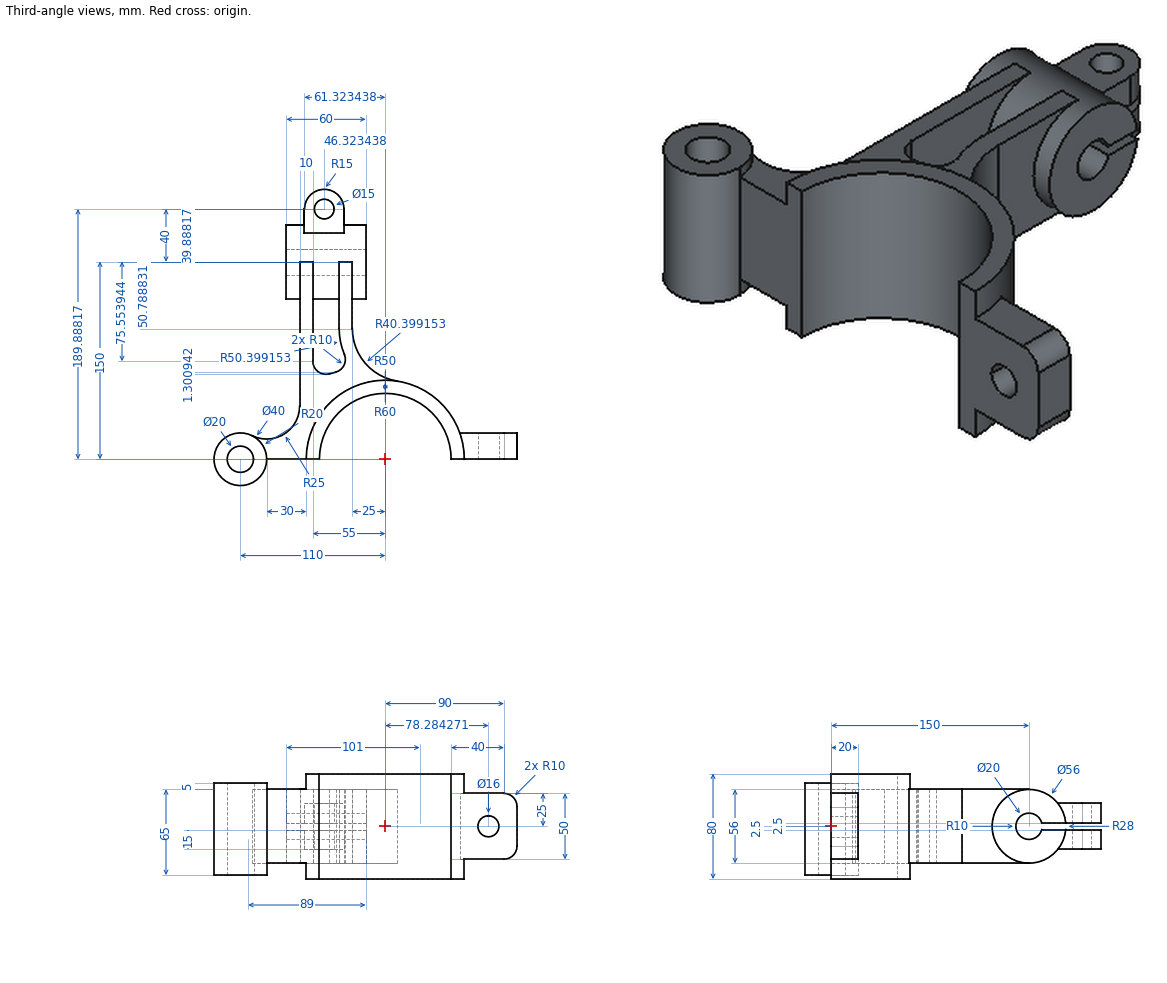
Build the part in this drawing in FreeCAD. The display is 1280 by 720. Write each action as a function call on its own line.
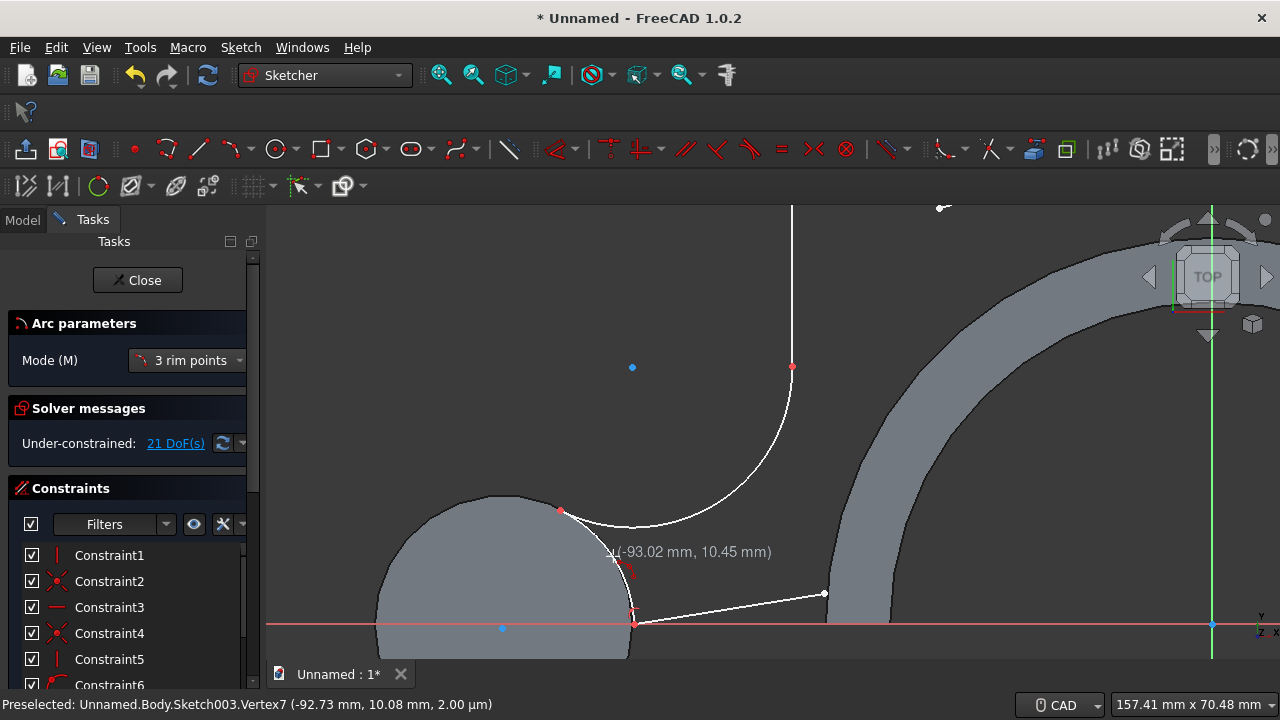
scroll(613, 557, down, 6)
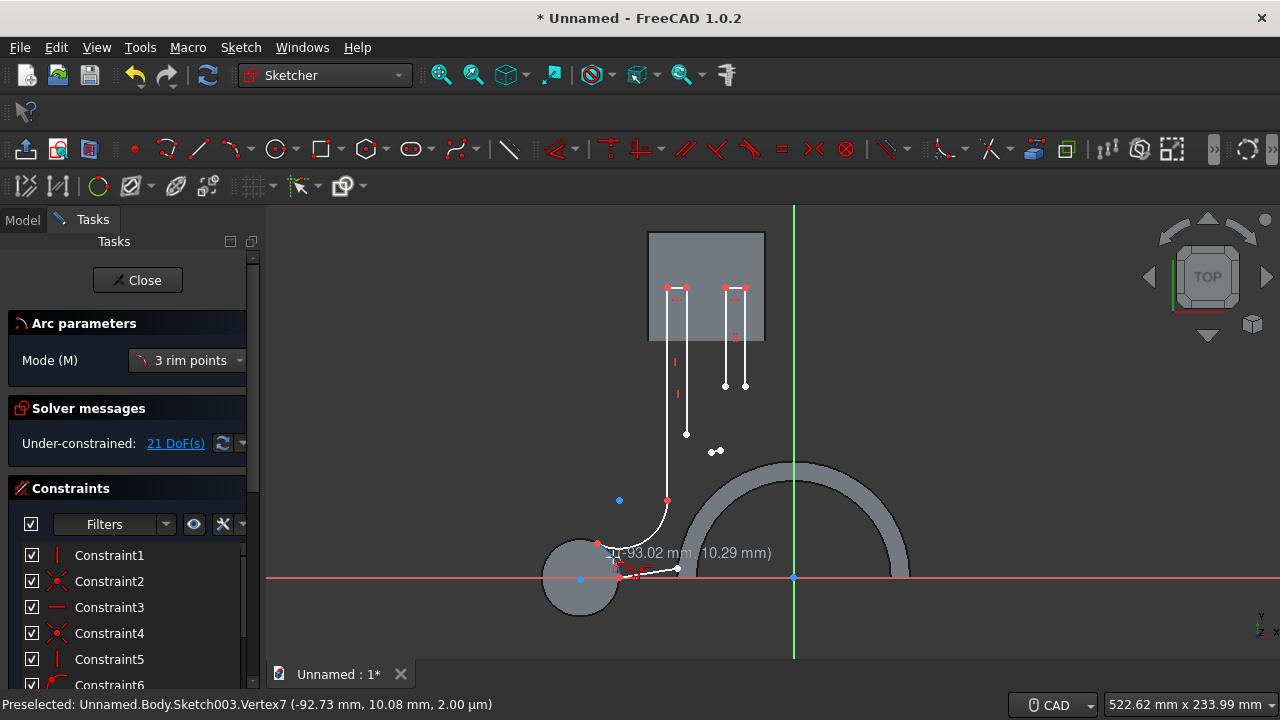
click(677, 569)
click(812, 463)
click(718, 489)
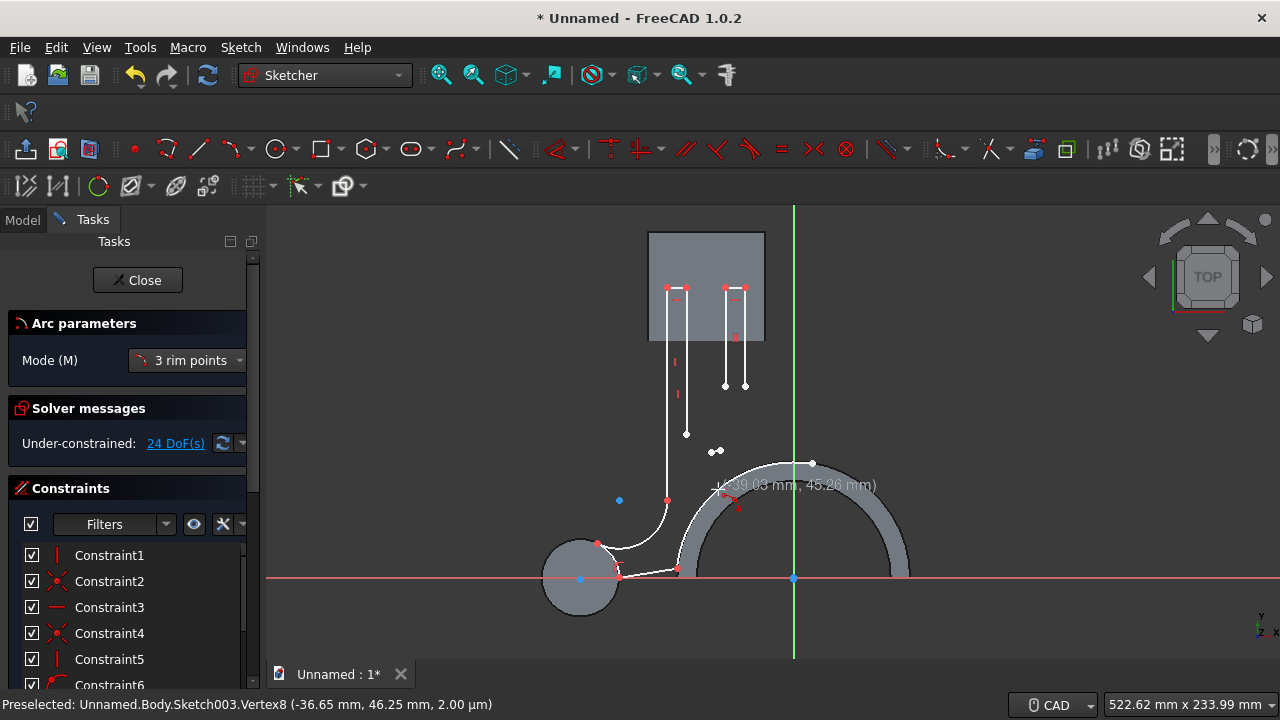
click(812, 464)
click(745, 387)
click(764, 436)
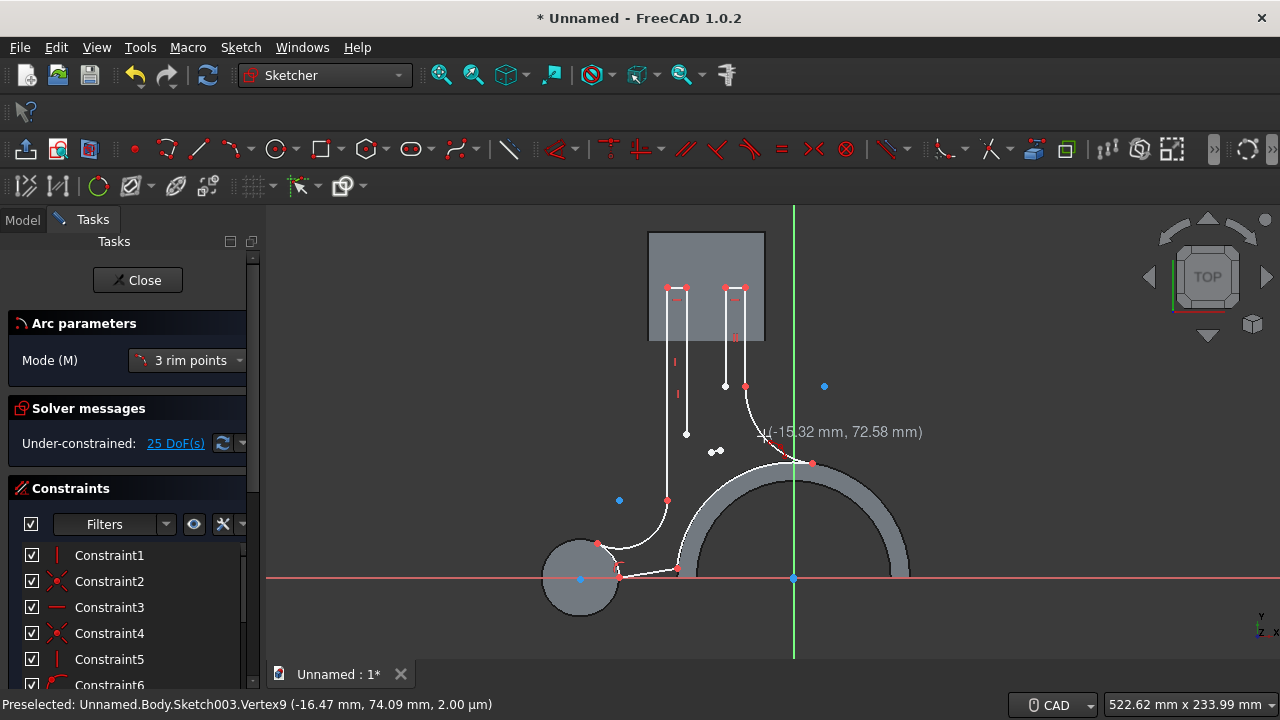
click(726, 387)
click(734, 423)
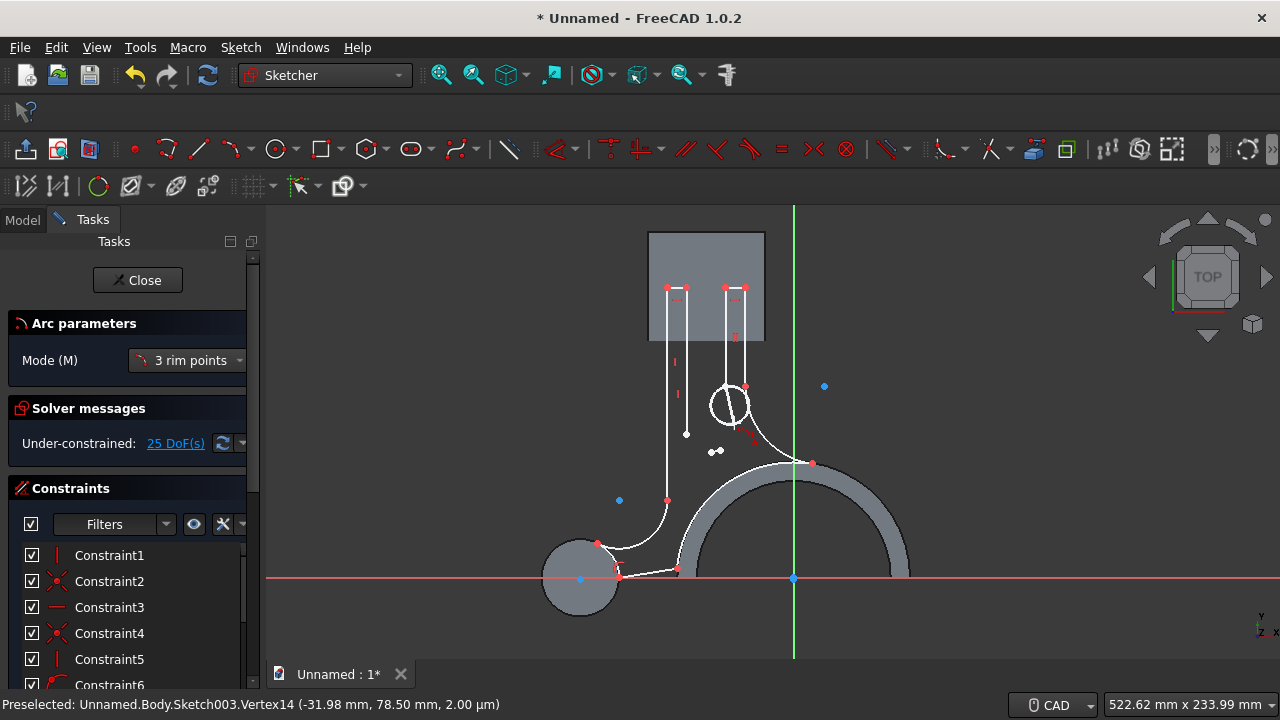
scroll(728, 405, up, 11)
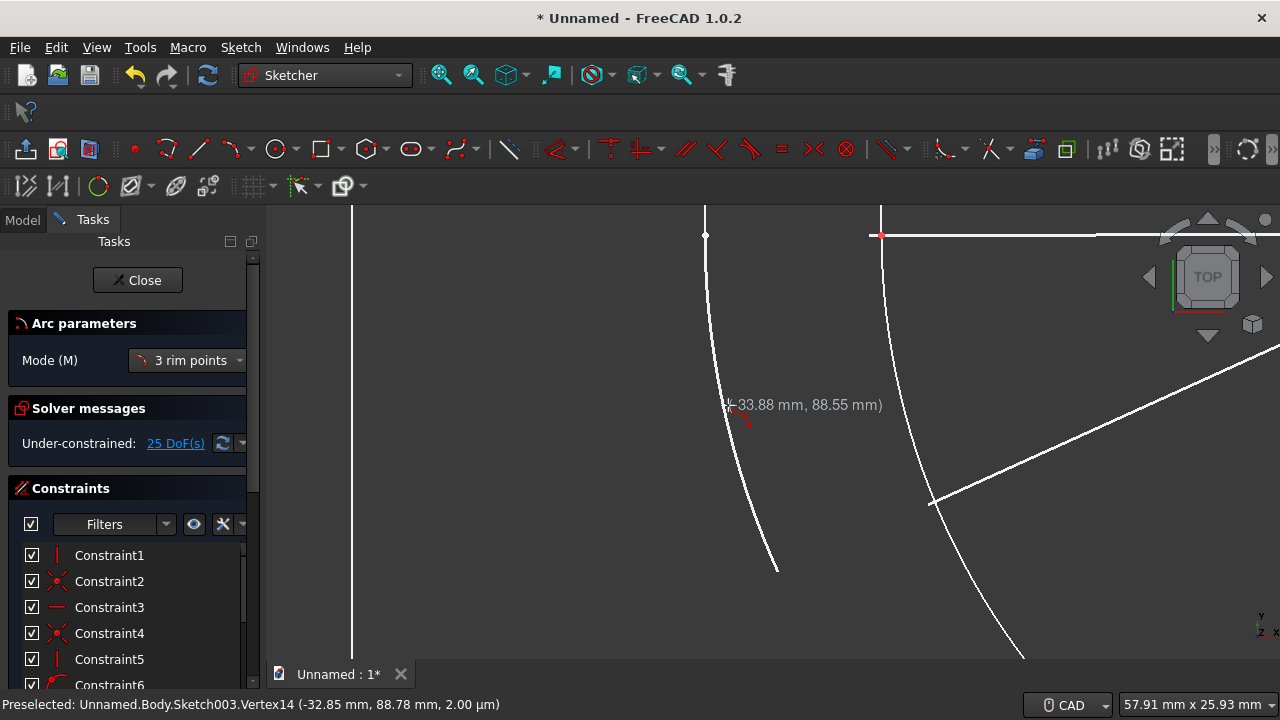
click(722, 399)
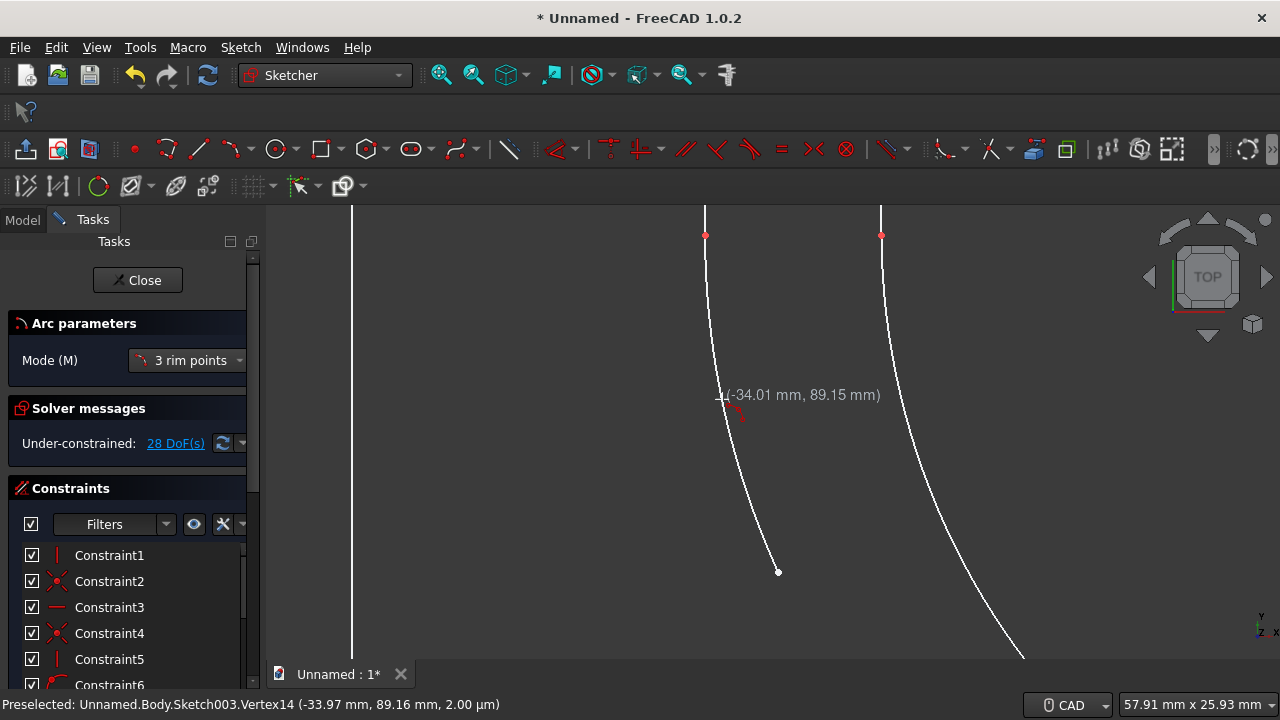
scroll(728, 405, down, 11)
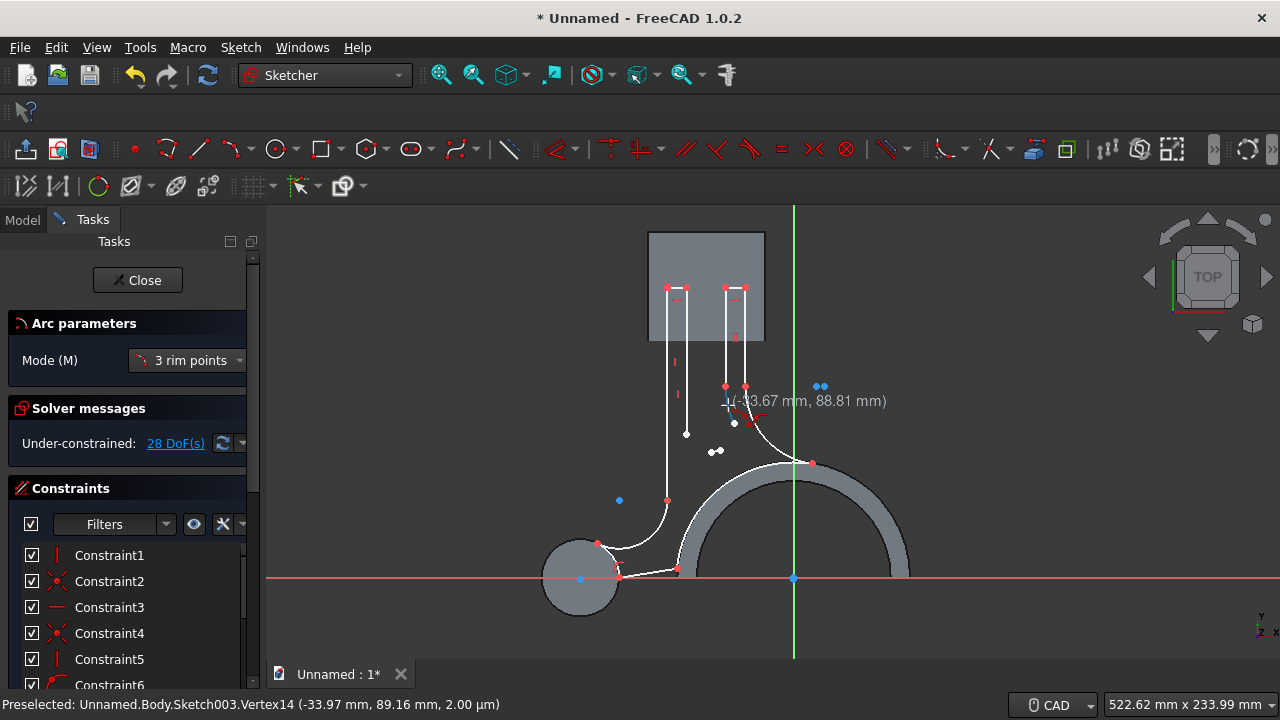
click(734, 424)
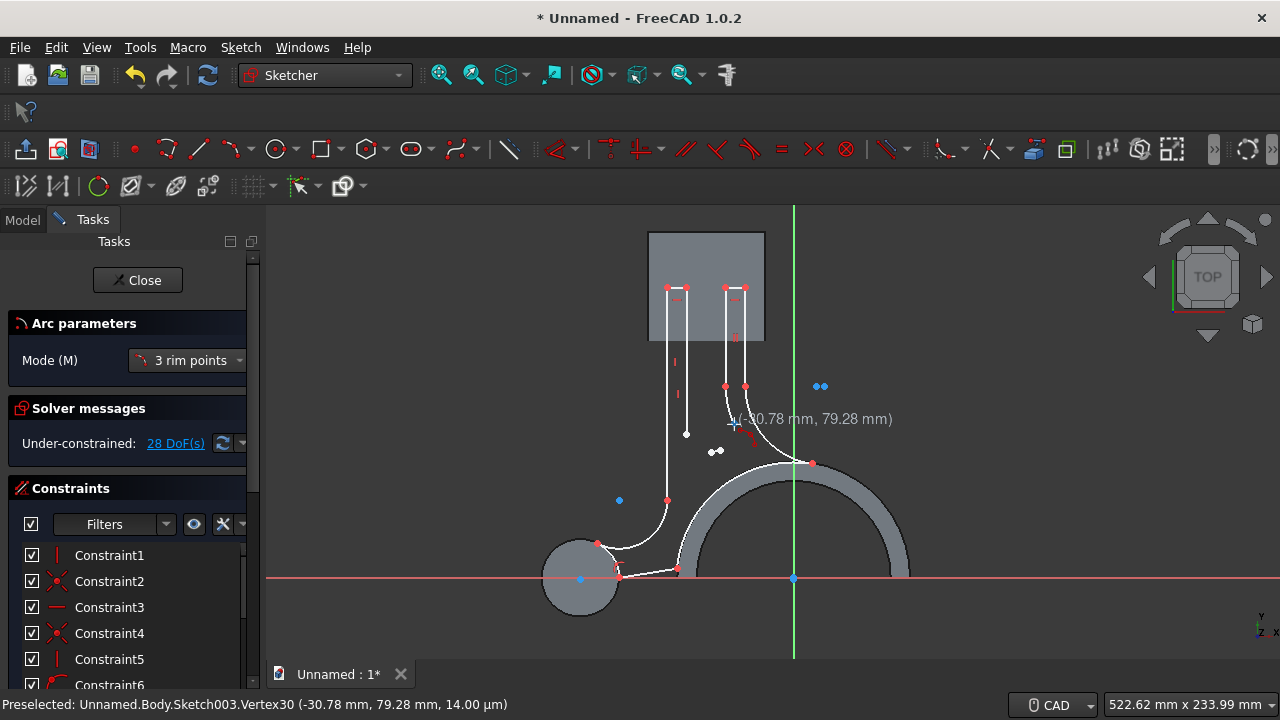
scroll(721, 450, up, 7)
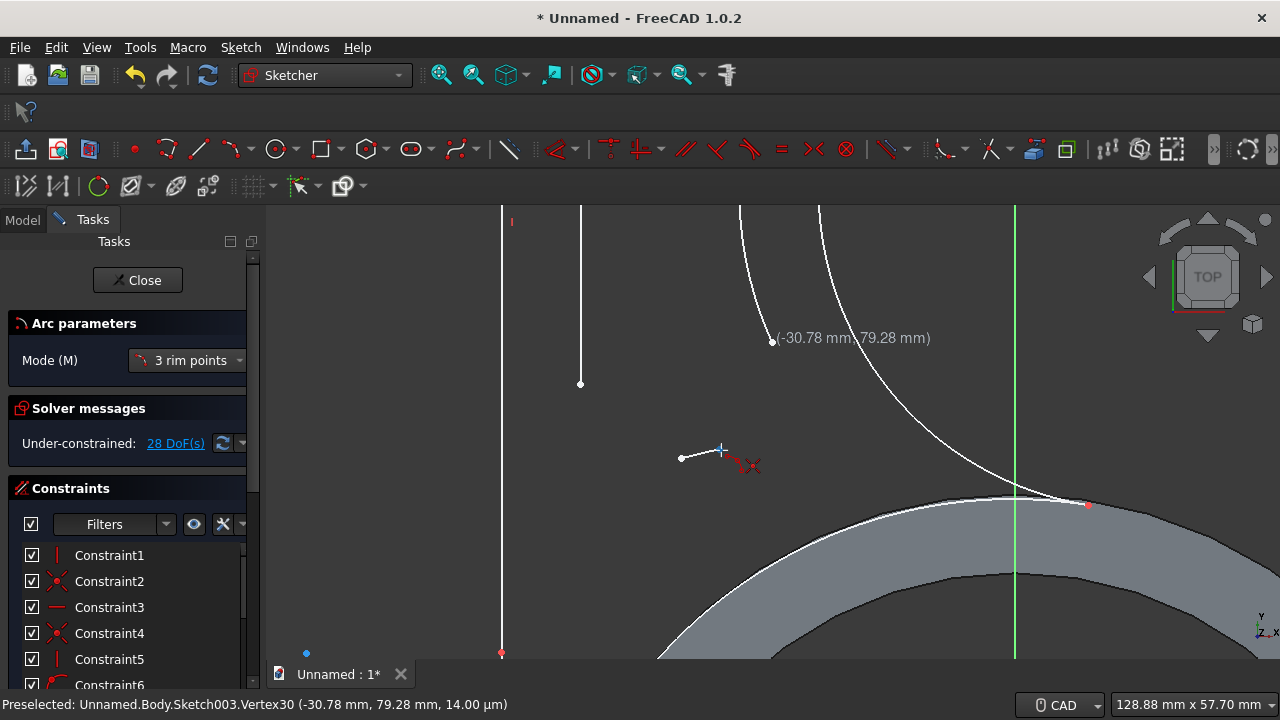
click(720, 449)
click(769, 405)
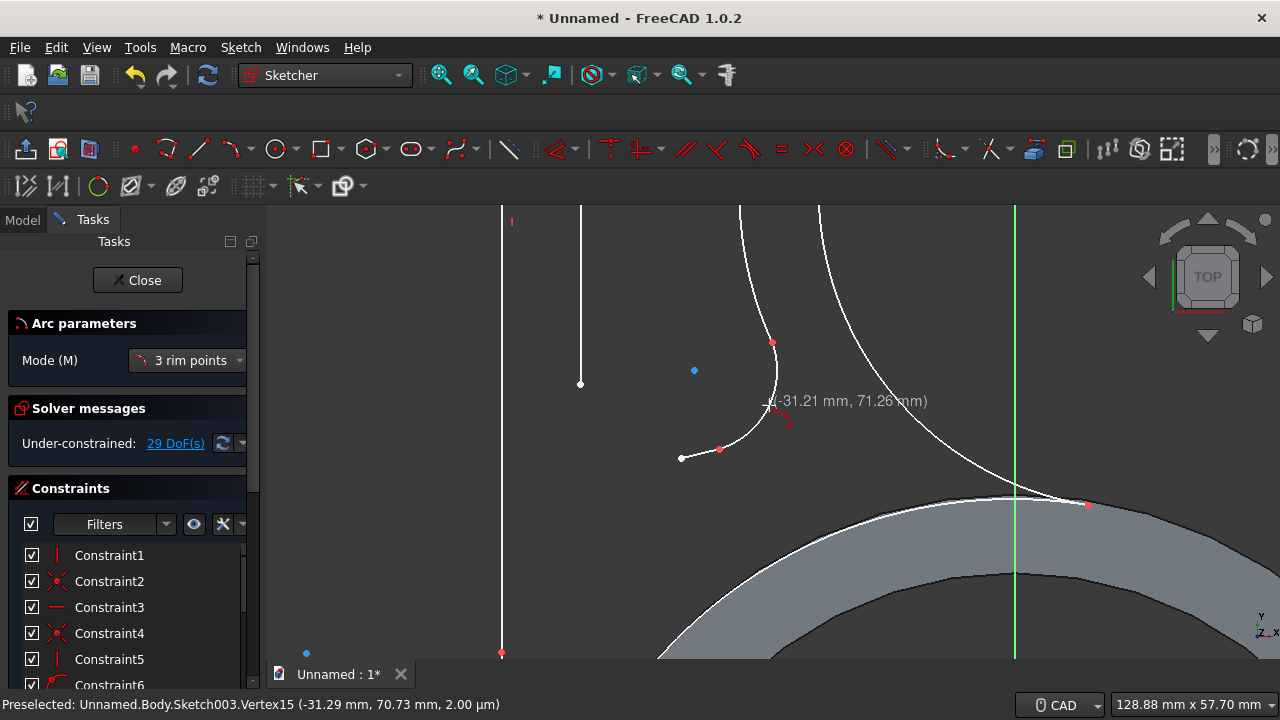
click(681, 458)